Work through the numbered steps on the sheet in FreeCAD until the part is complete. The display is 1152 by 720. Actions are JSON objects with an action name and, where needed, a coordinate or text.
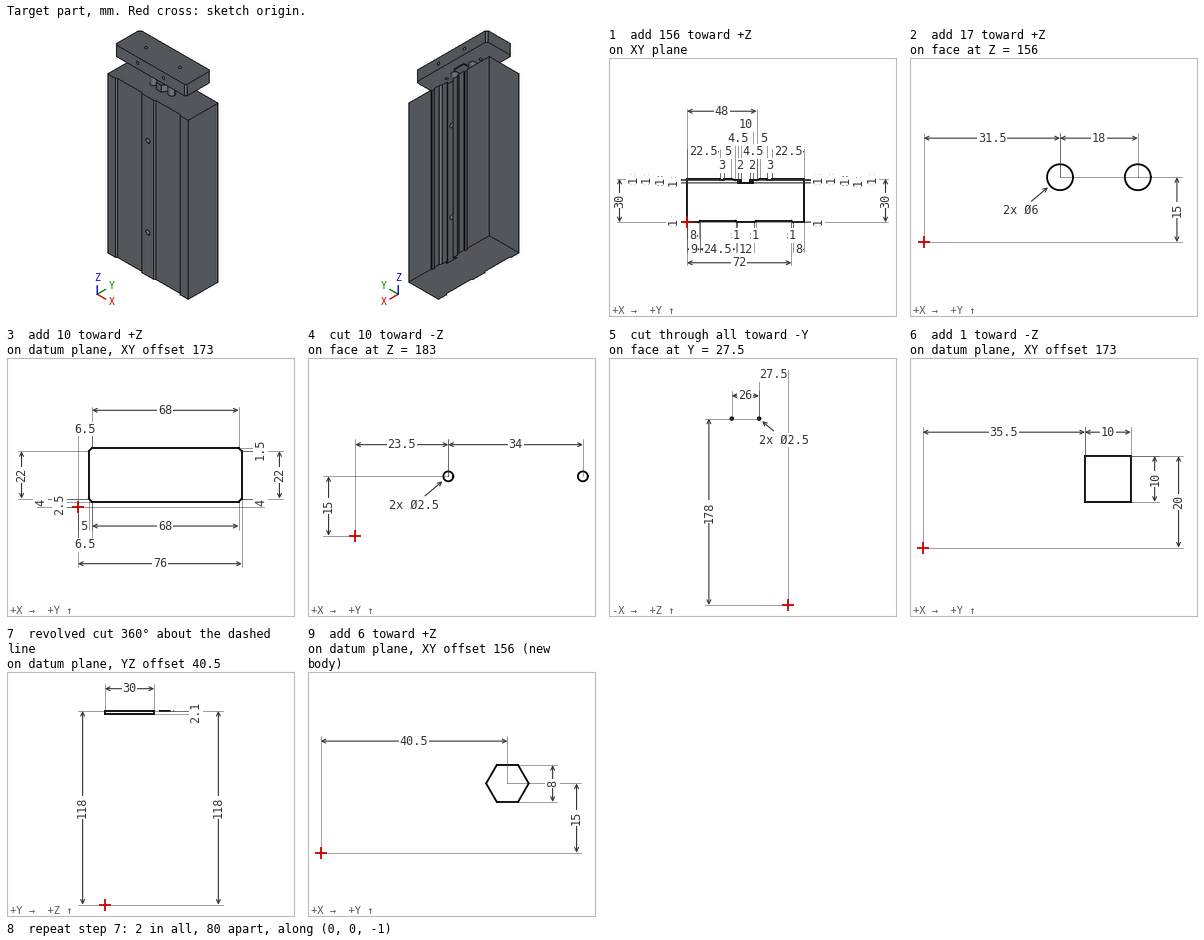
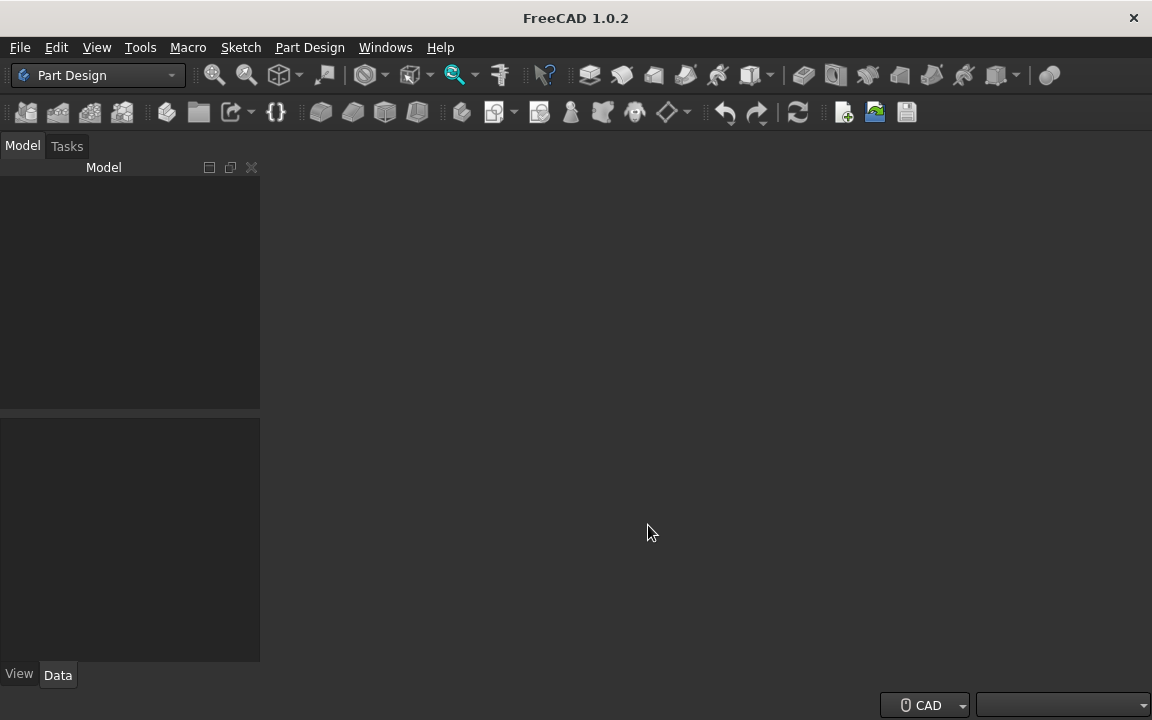
{"action": "key", "text": "ctrl+n"}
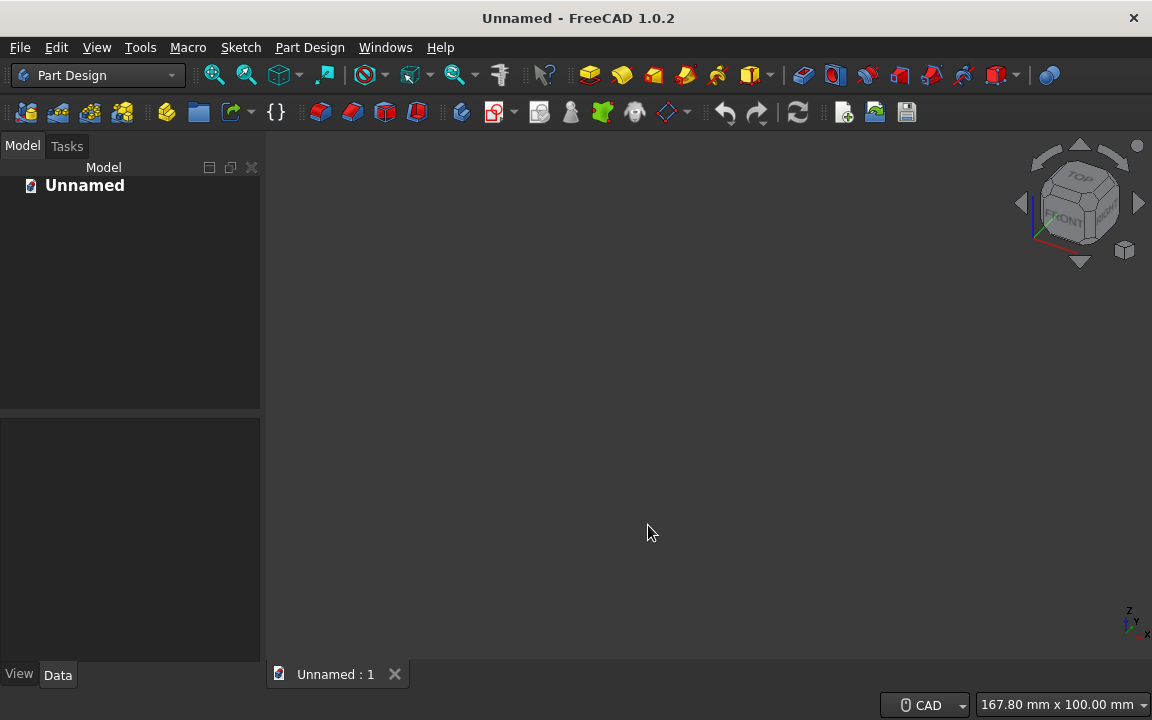
{"action": "left_click", "coordinate": [494, 112]}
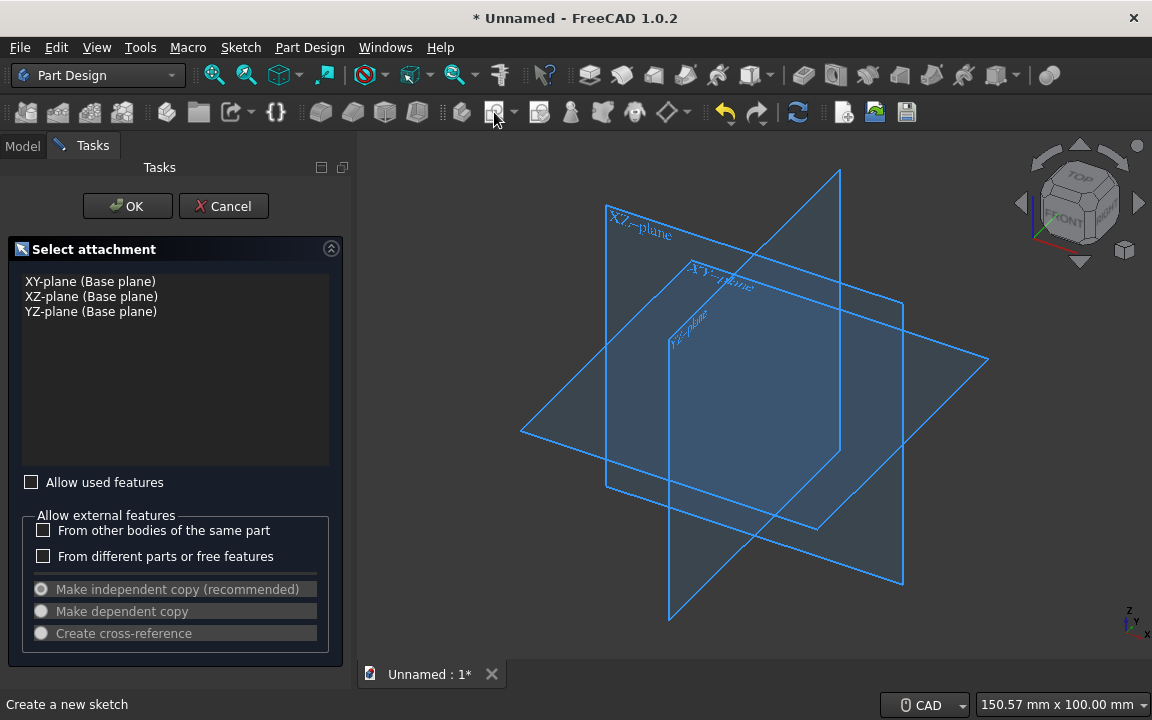
{"action": "left_click", "coordinate": [82, 282]}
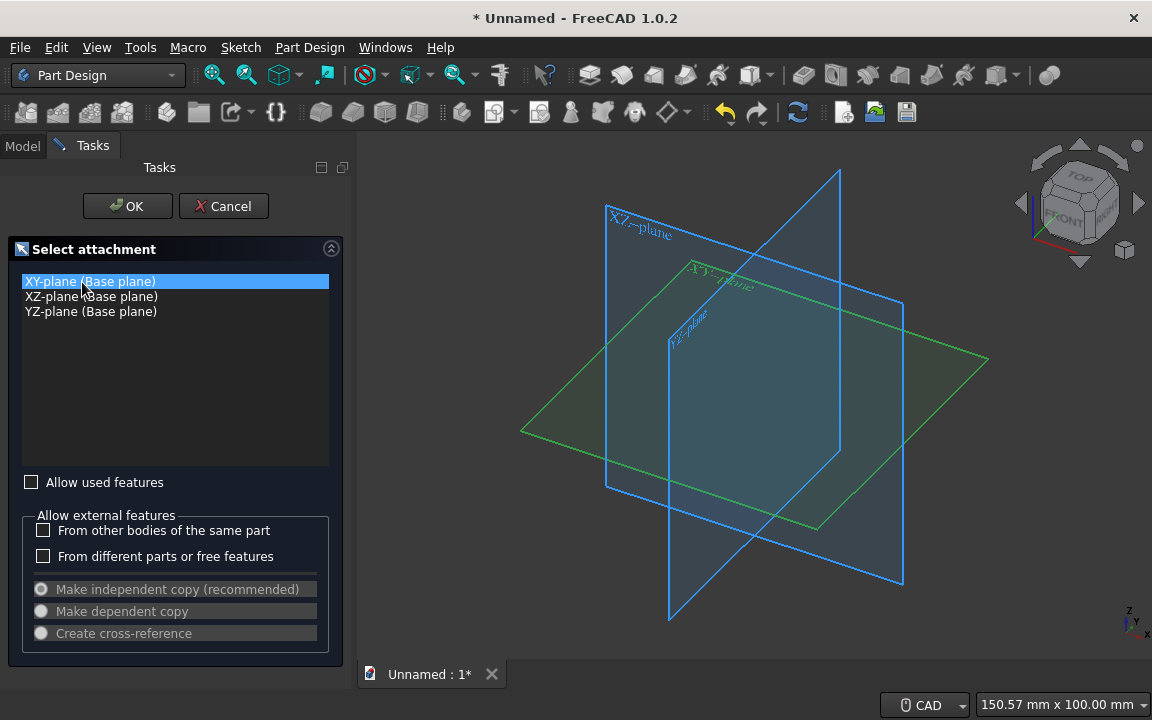
{"action": "left_click", "coordinate": [128, 206]}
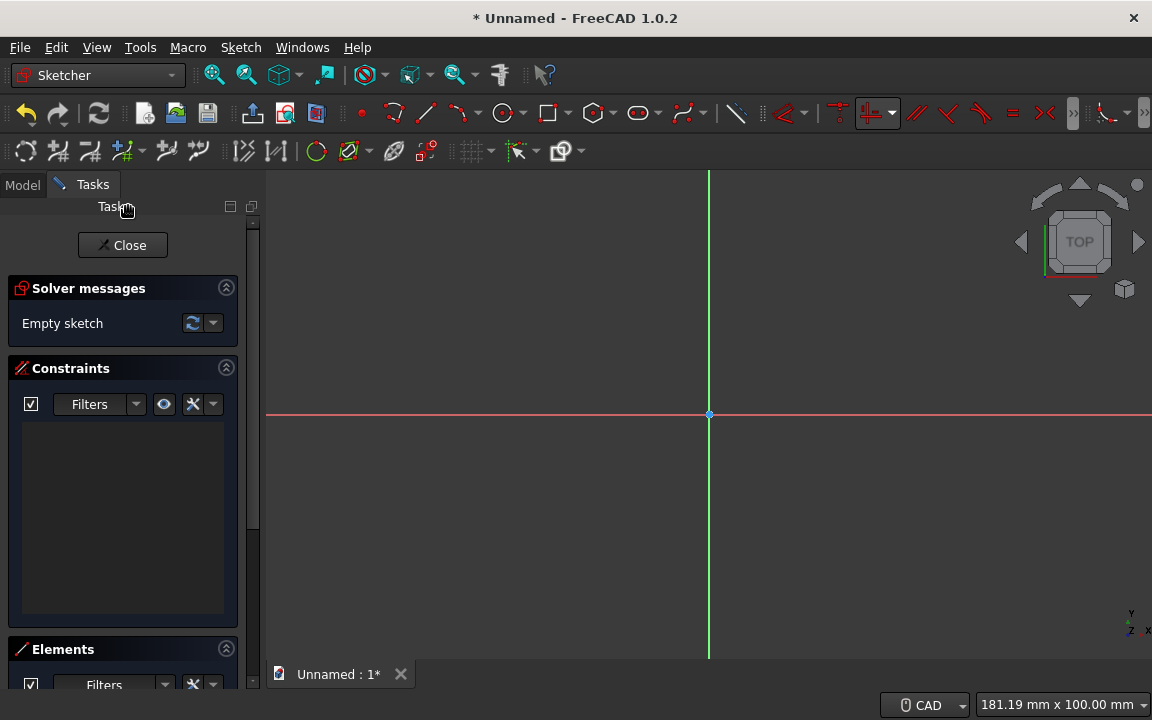
{"action": "scroll", "coordinate": [294, 631], "scroll_direction": "down", "scroll_amount": 1}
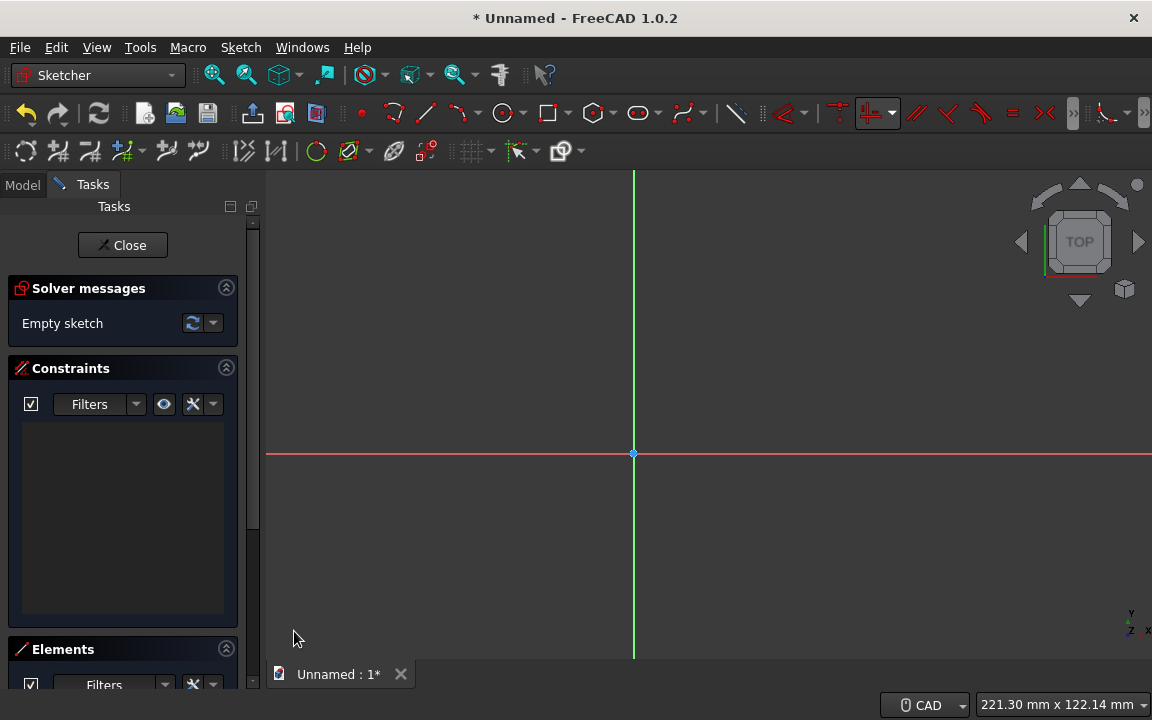
{"action": "scroll", "coordinate": [987, 352], "scroll_direction": "up", "scroll_amount": 2}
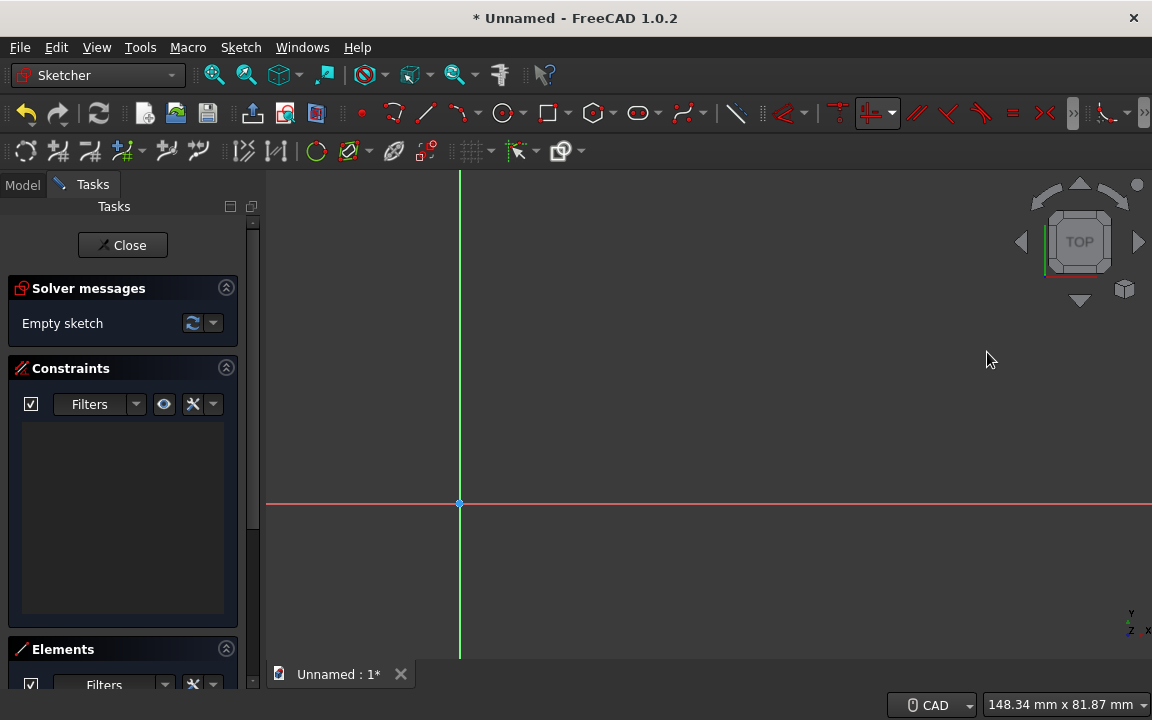
{"action": "left_click", "coordinate": [394, 114]}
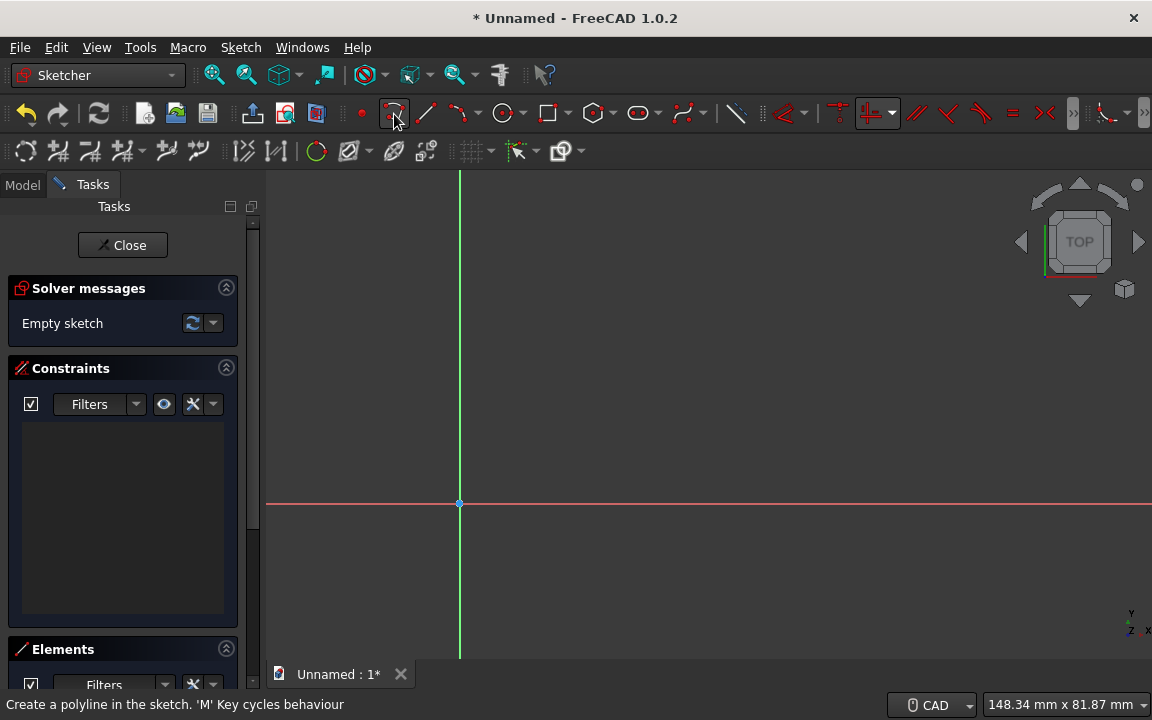
{"action": "left_click", "coordinate": [460, 504]}
{"action": "left_click", "coordinate": [507, 495]}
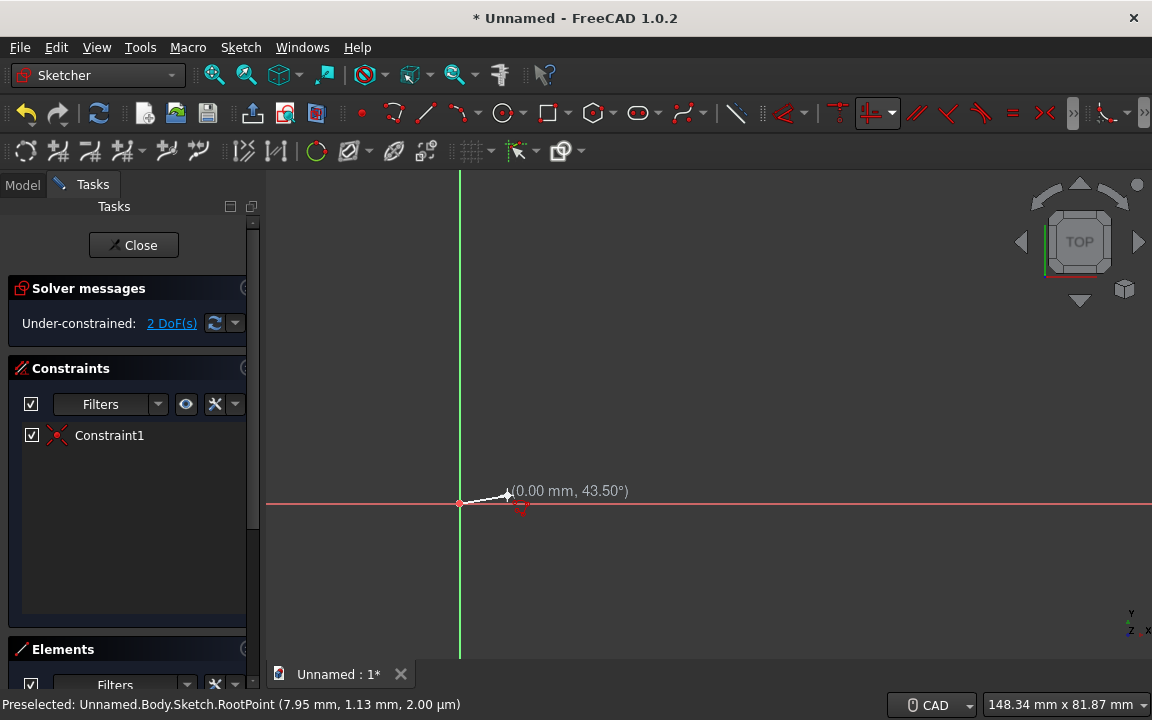
{"action": "scroll", "coordinate": [513, 498], "scroll_direction": "up", "scroll_amount": 5}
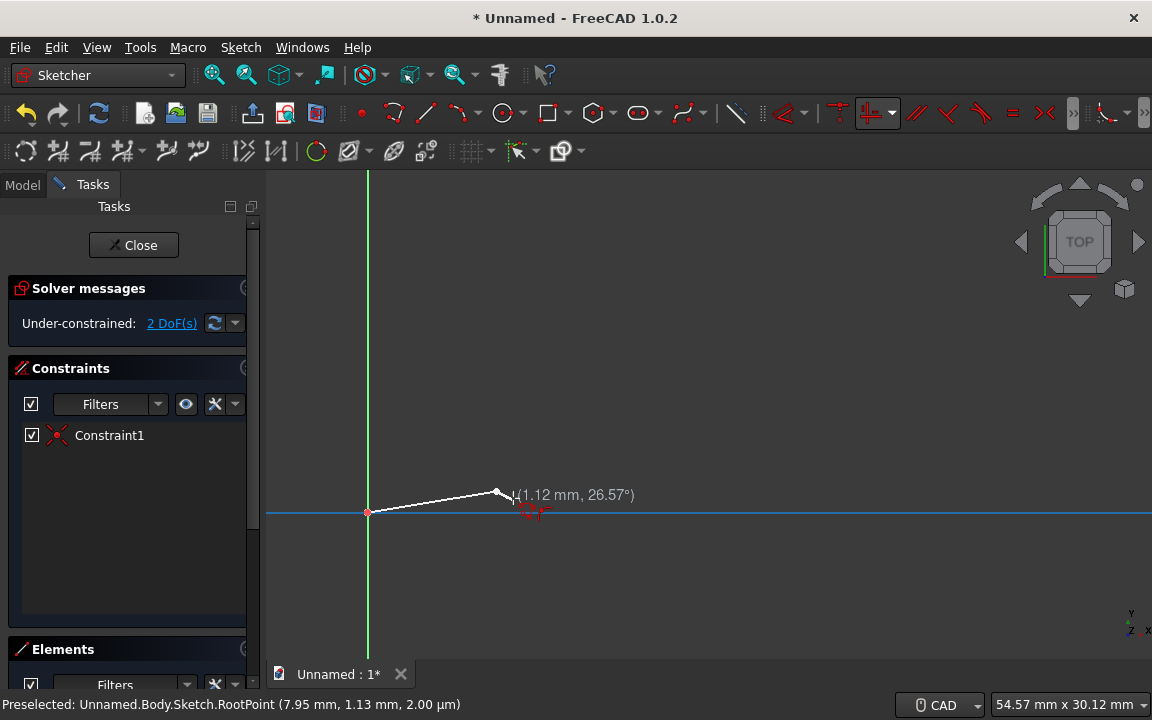
{"action": "left_click", "coordinate": [514, 497]}
{"action": "left_click", "coordinate": [911, 497]}
{"action": "left_click", "coordinate": [928, 513]}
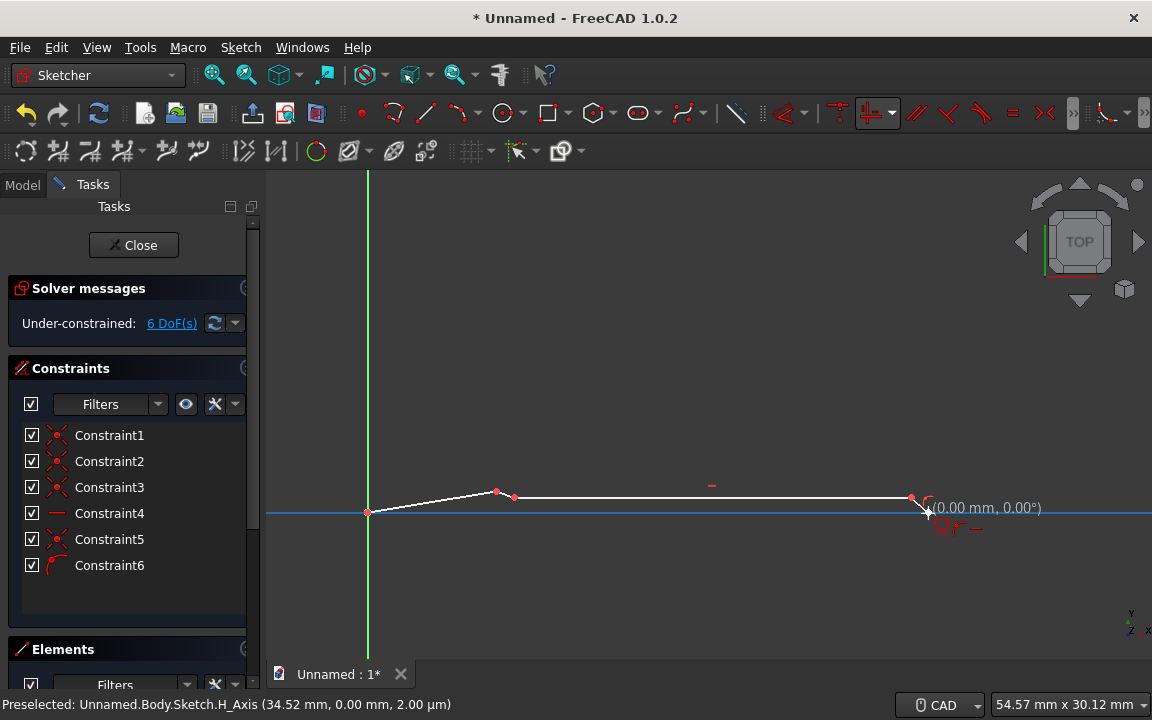
{"action": "scroll", "coordinate": [417, 499], "scroll_direction": "down", "scroll_amount": 5}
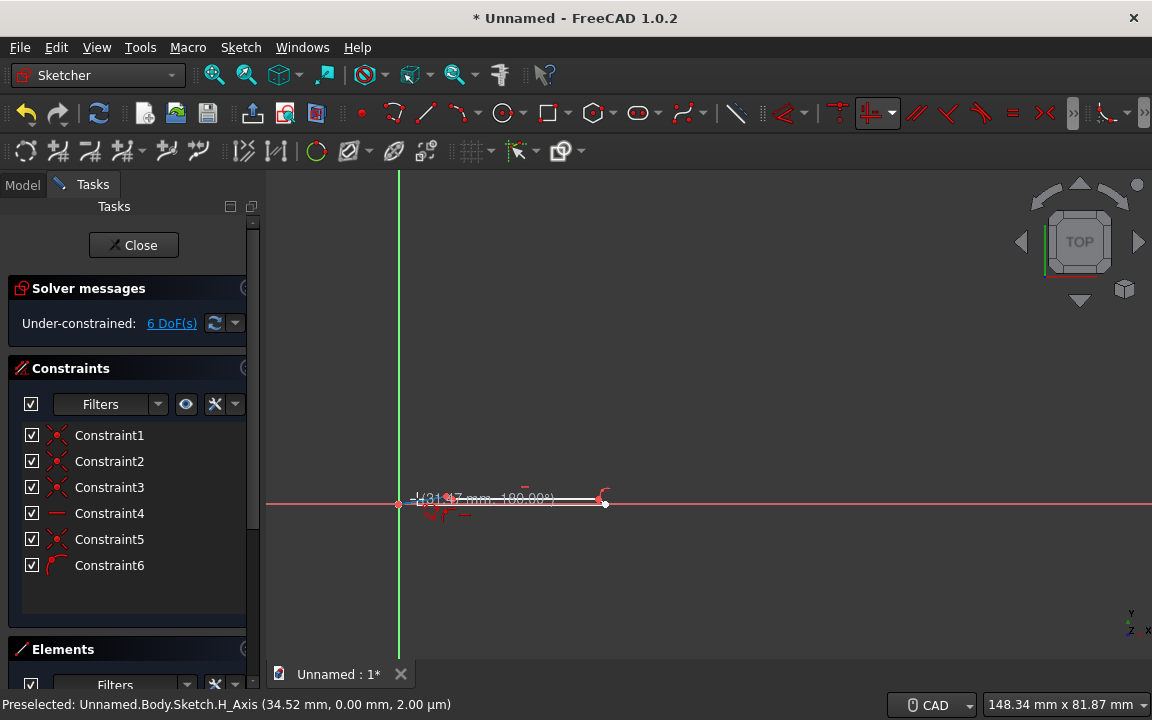
{"action": "left_click", "coordinate": [677, 495]}